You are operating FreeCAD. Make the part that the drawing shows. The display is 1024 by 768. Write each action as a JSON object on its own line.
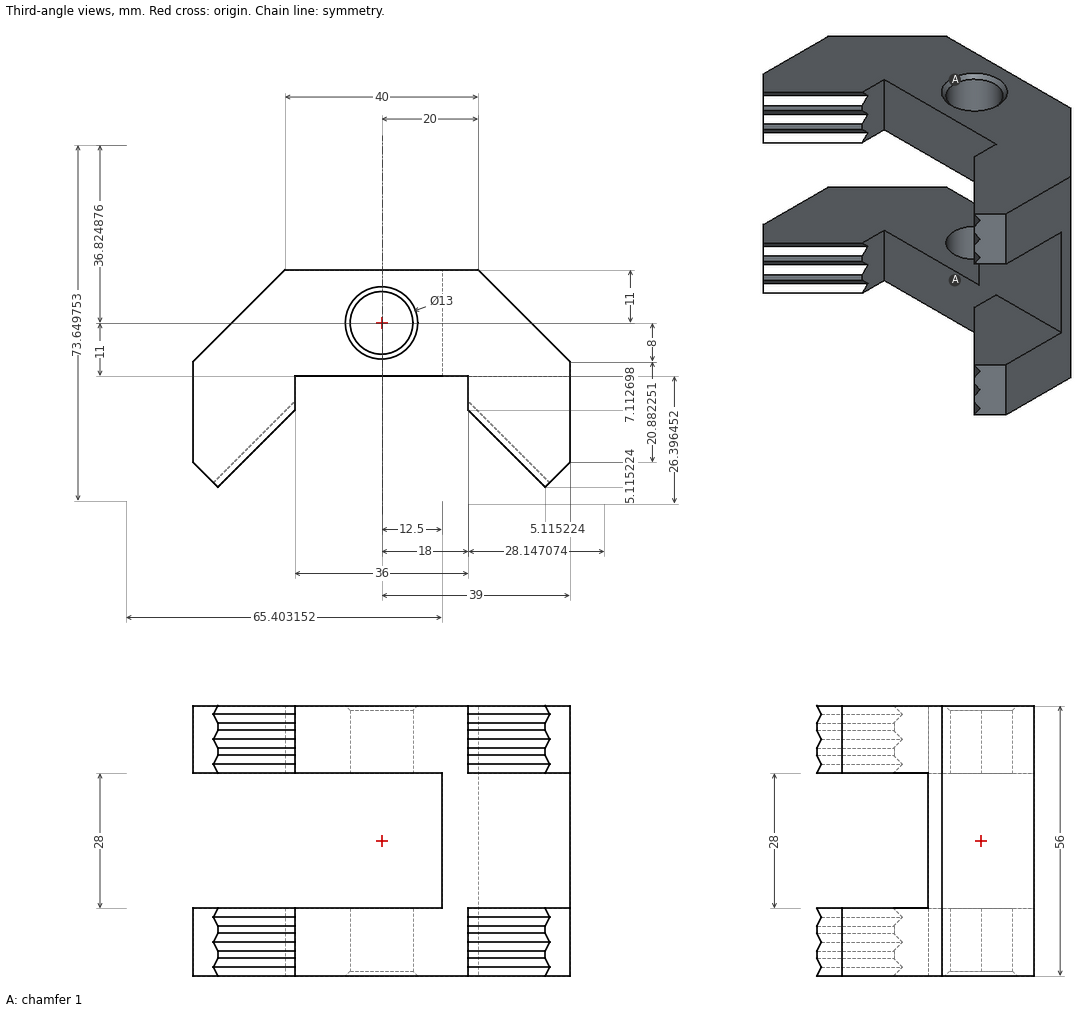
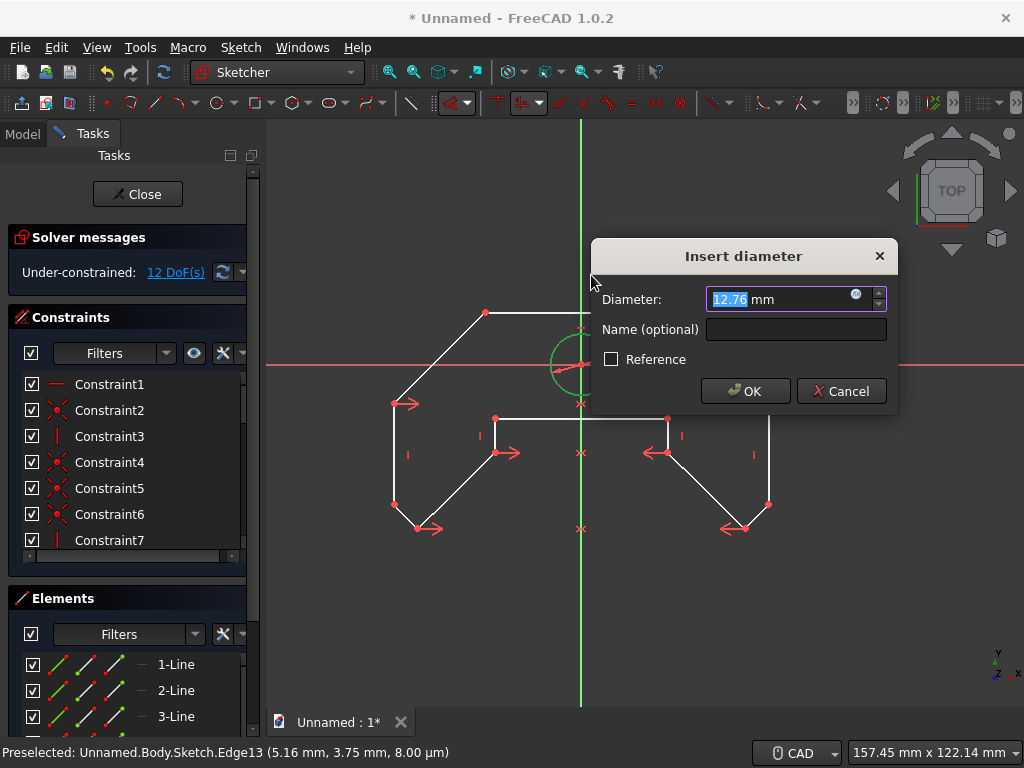
{"action": "type", "text": "13"}
{"action": "key", "text": "Return"}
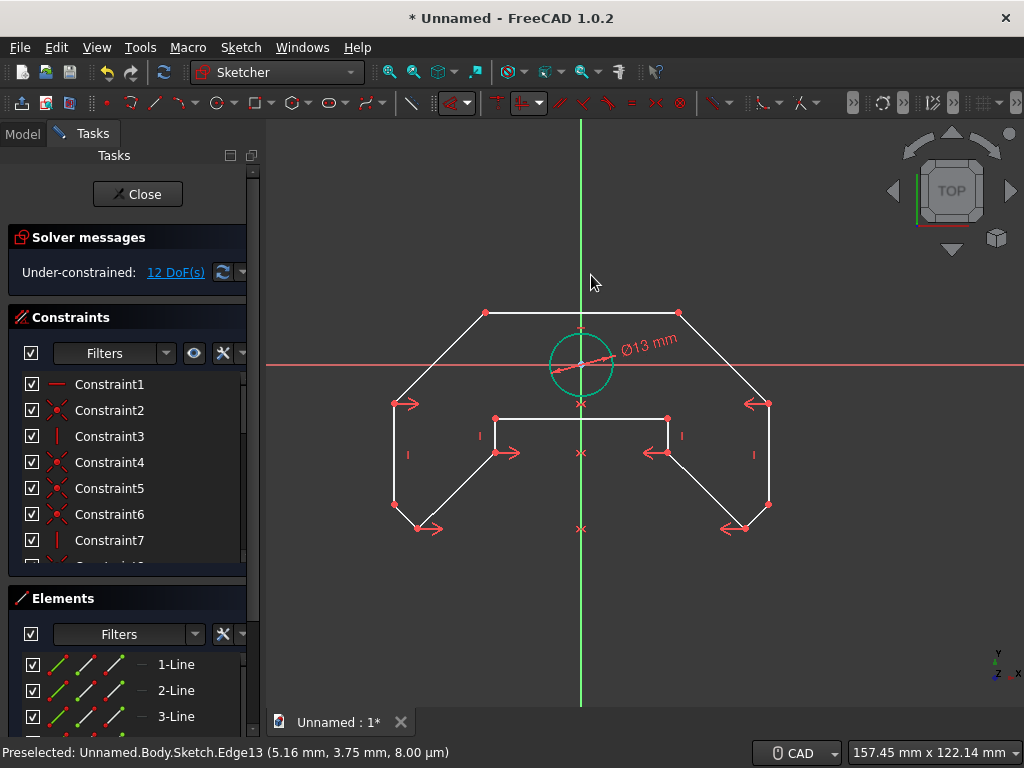
{"action": "left_click", "coordinate": [547, 419]}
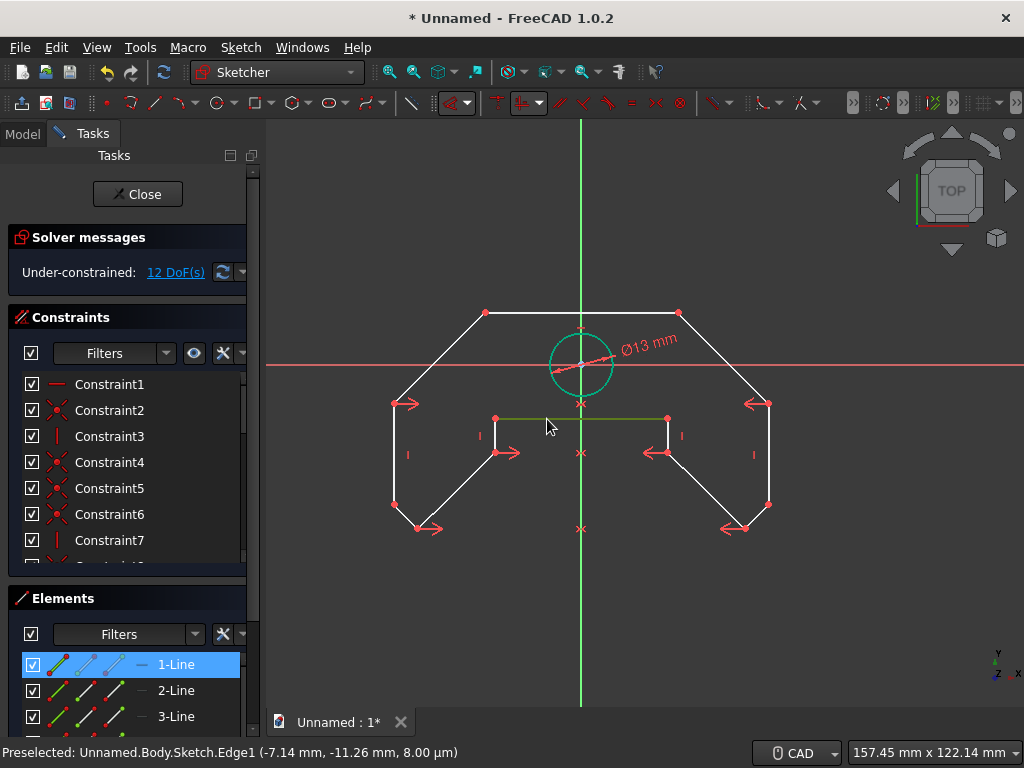
{"action": "key", "text": "l"}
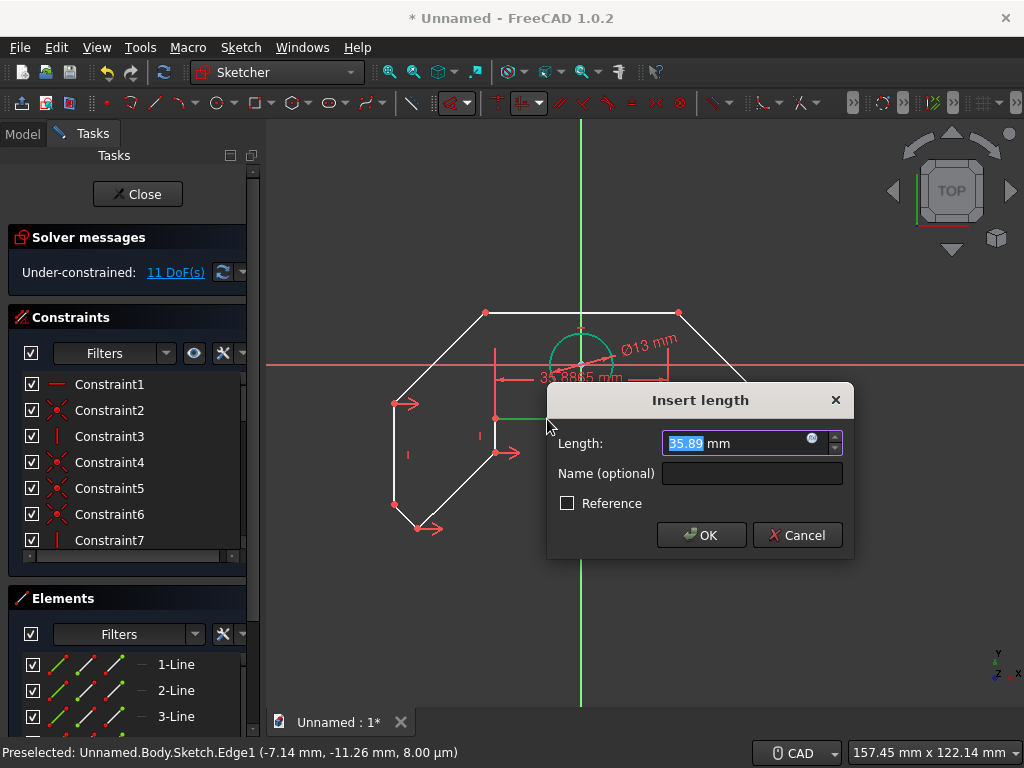
{"action": "type", "text": "36"}
{"action": "key", "text": "Return"}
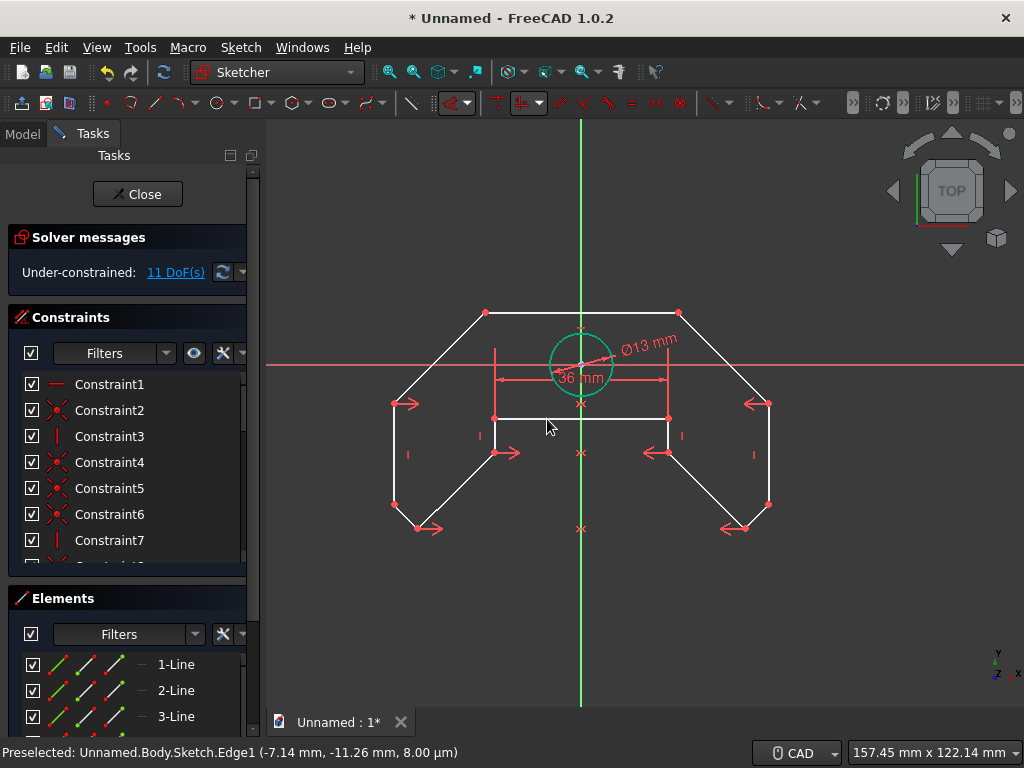
{"action": "left_click", "coordinate": [620, 313]}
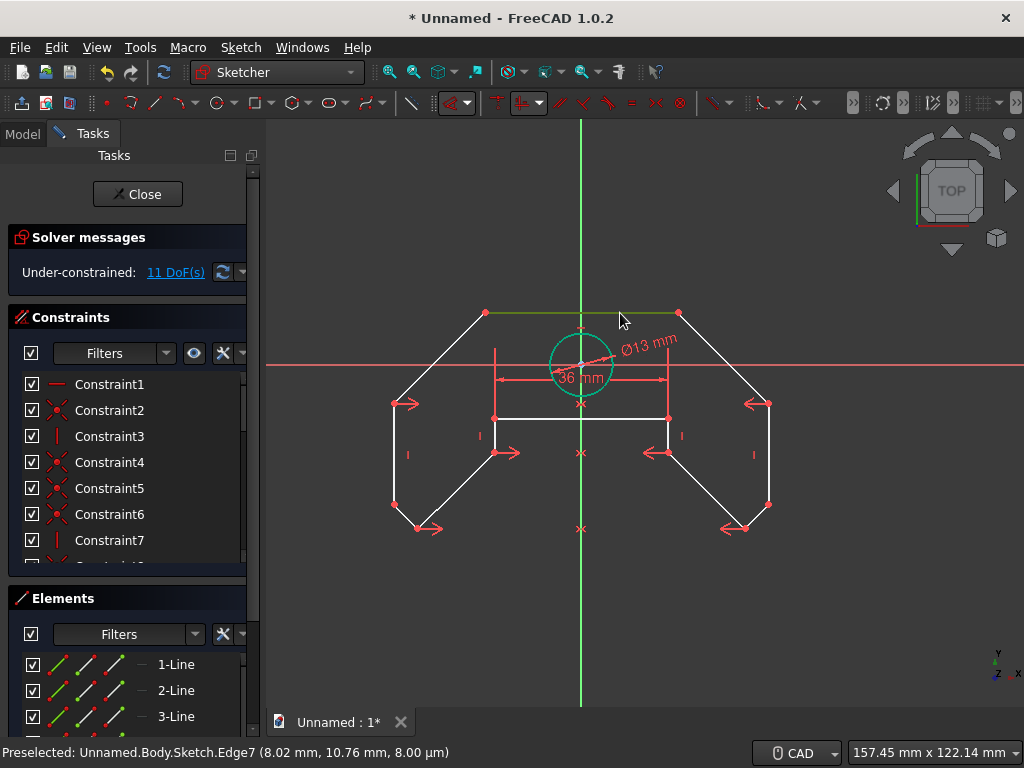
{"action": "key", "text": "l"}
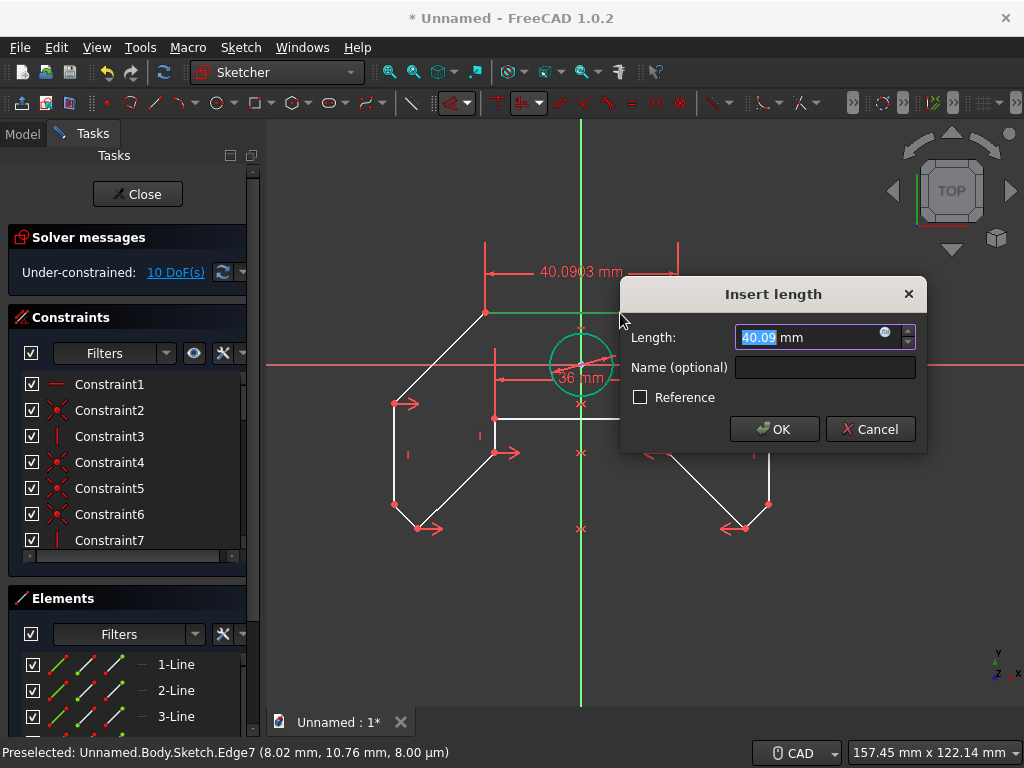
{"action": "type", "text": "40"}
{"action": "key", "text": "Return"}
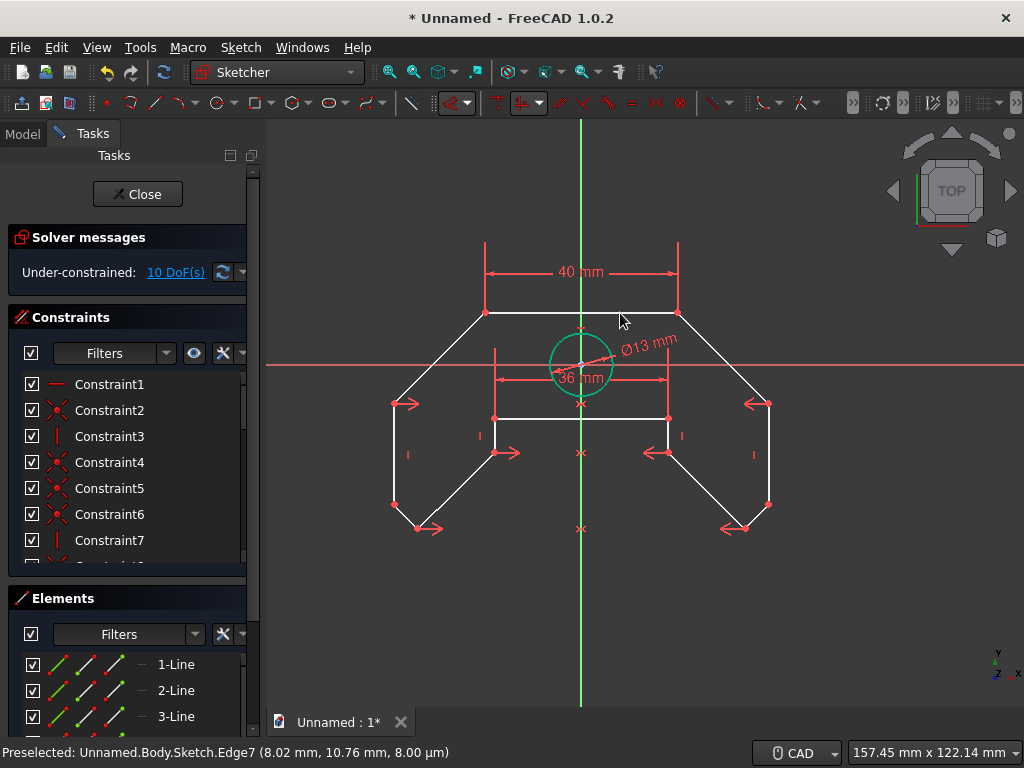
{"action": "left_click", "coordinate": [769, 404]}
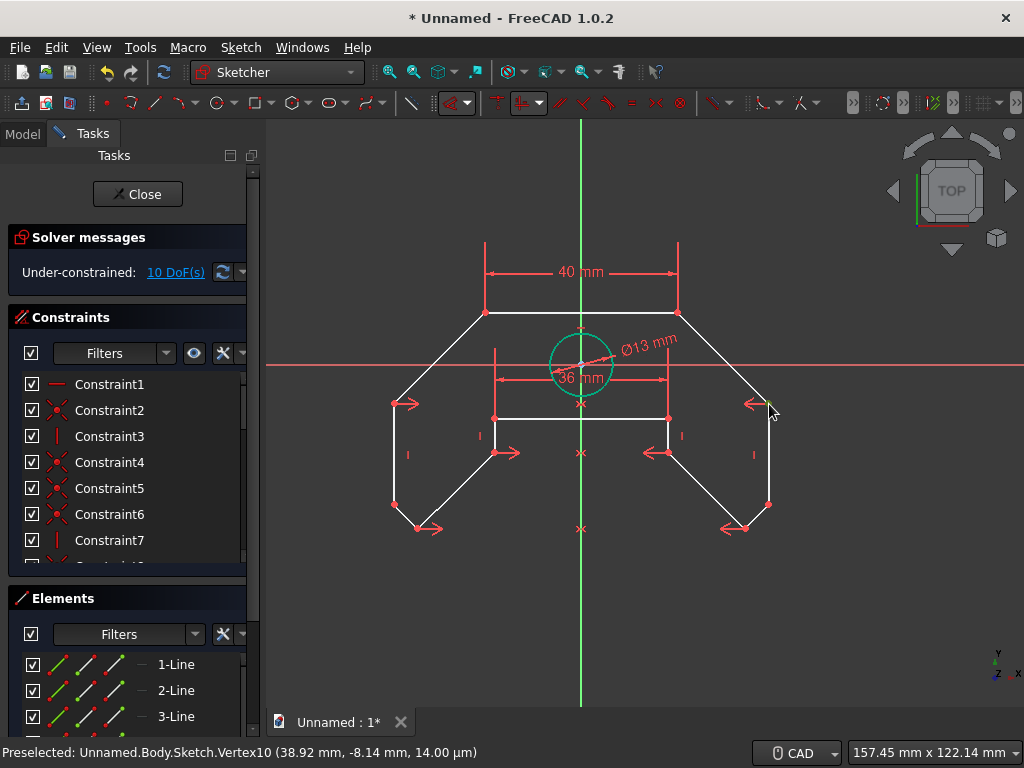
{"action": "left_click", "coordinate": [470, 104]}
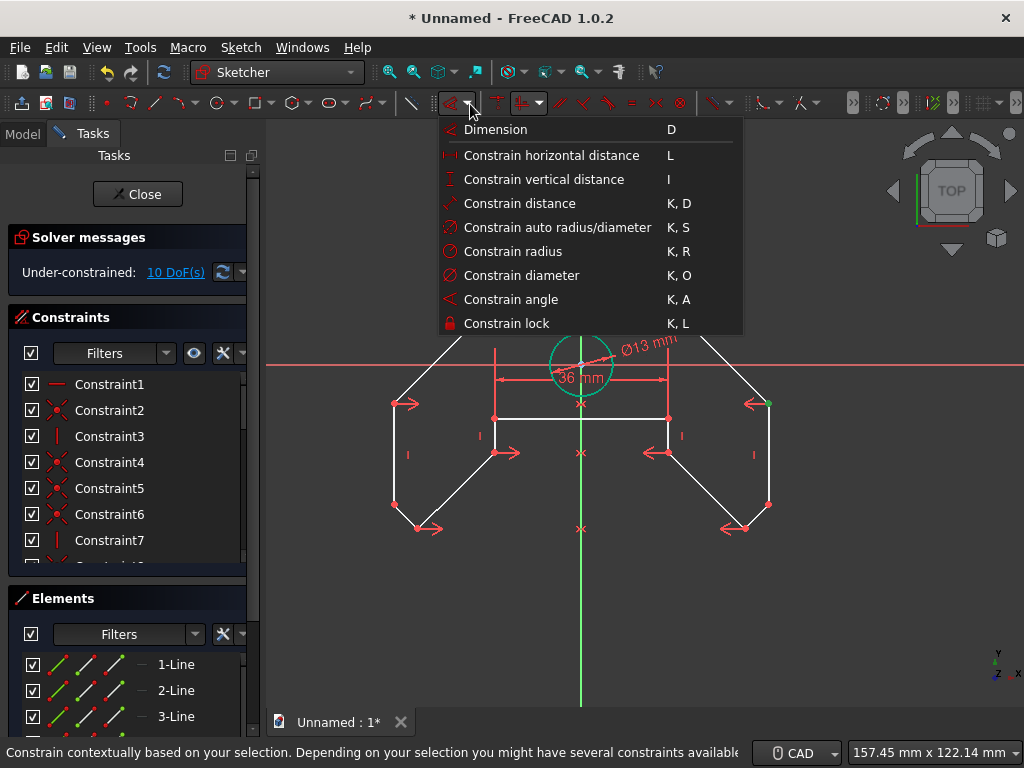
{"action": "left_click", "coordinate": [591, 179]}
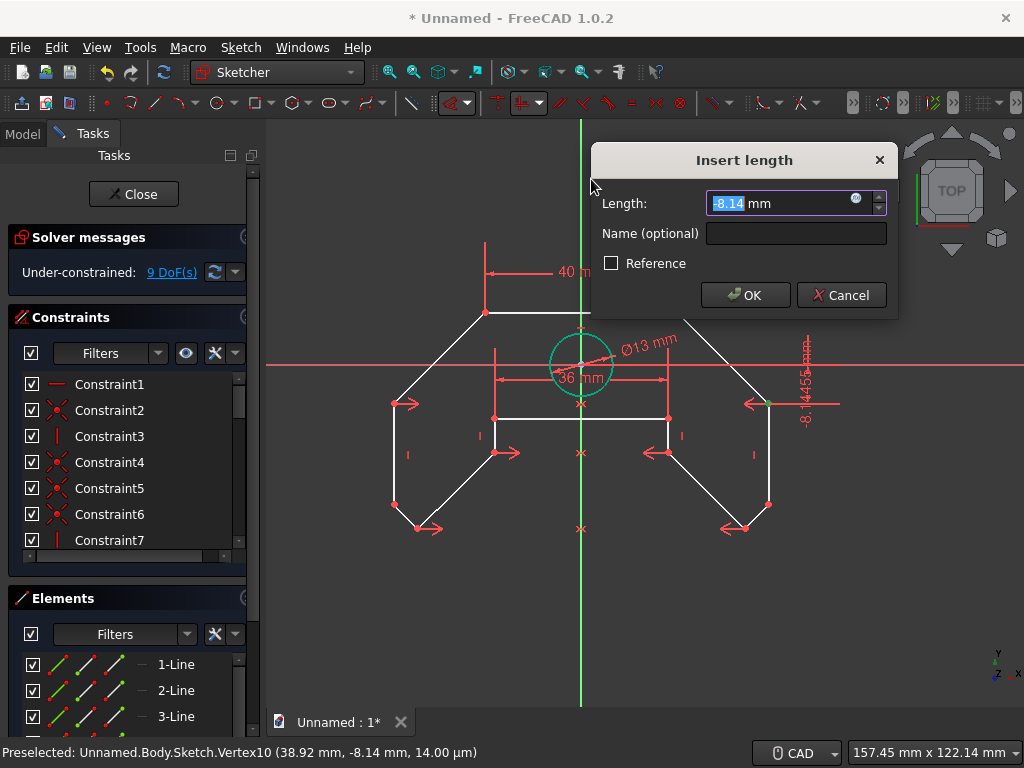
{"action": "type", "text": "-8"}
{"action": "key", "text": "Return"}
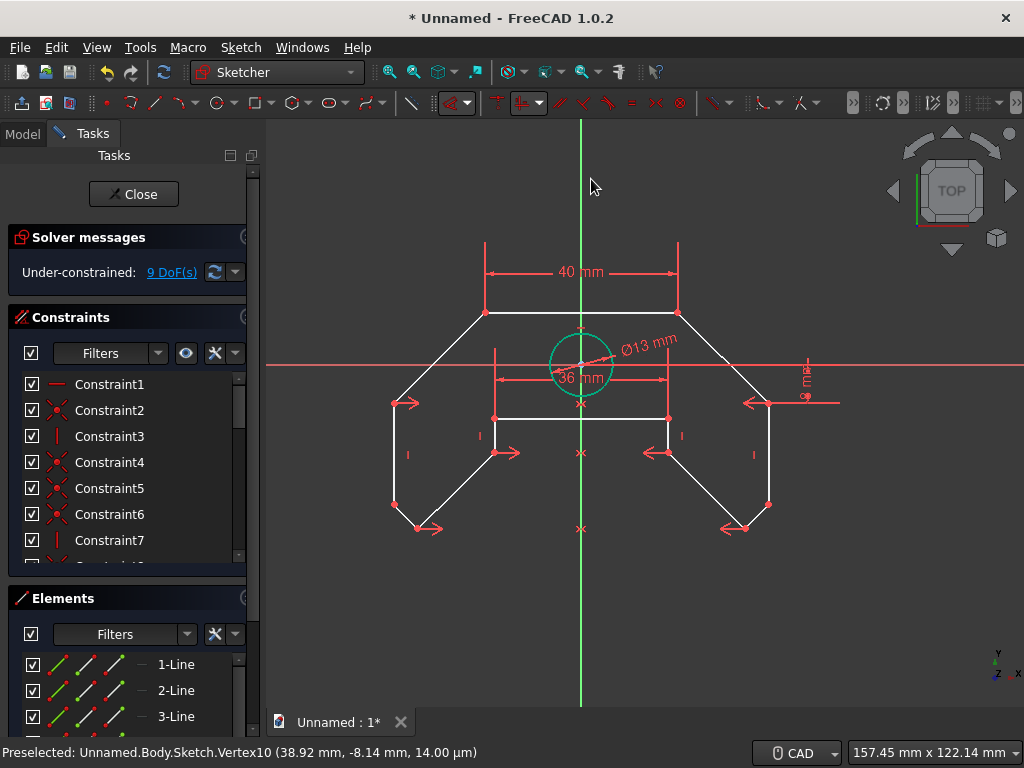
{"action": "left_click", "coordinate": [495, 419]}